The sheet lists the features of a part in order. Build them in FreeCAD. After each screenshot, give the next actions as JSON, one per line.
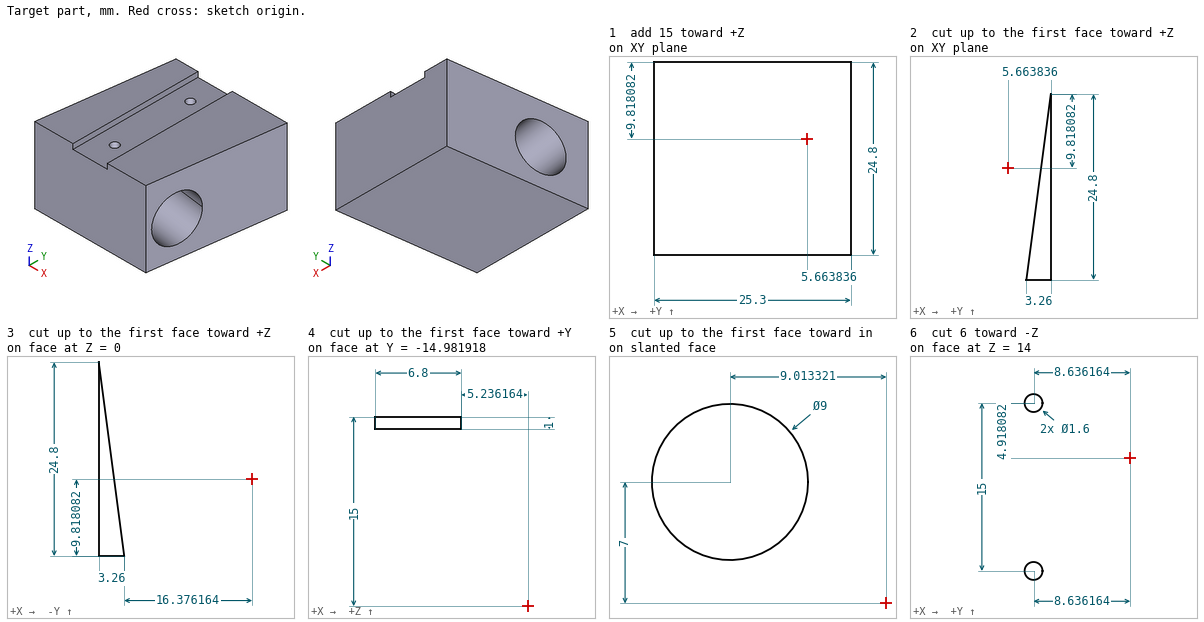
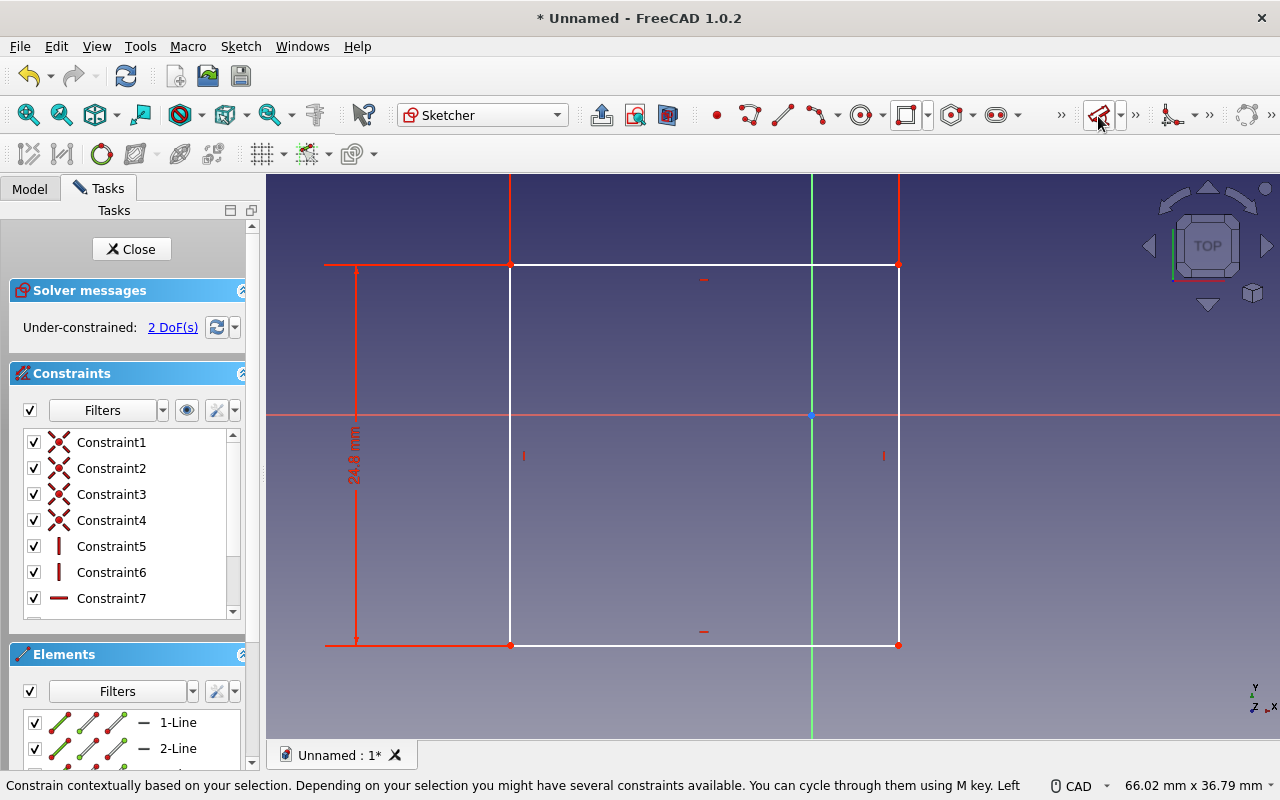
{"action": "left_click", "coordinate": [510, 265]}
{"action": "left_click", "coordinate": [476, 340]}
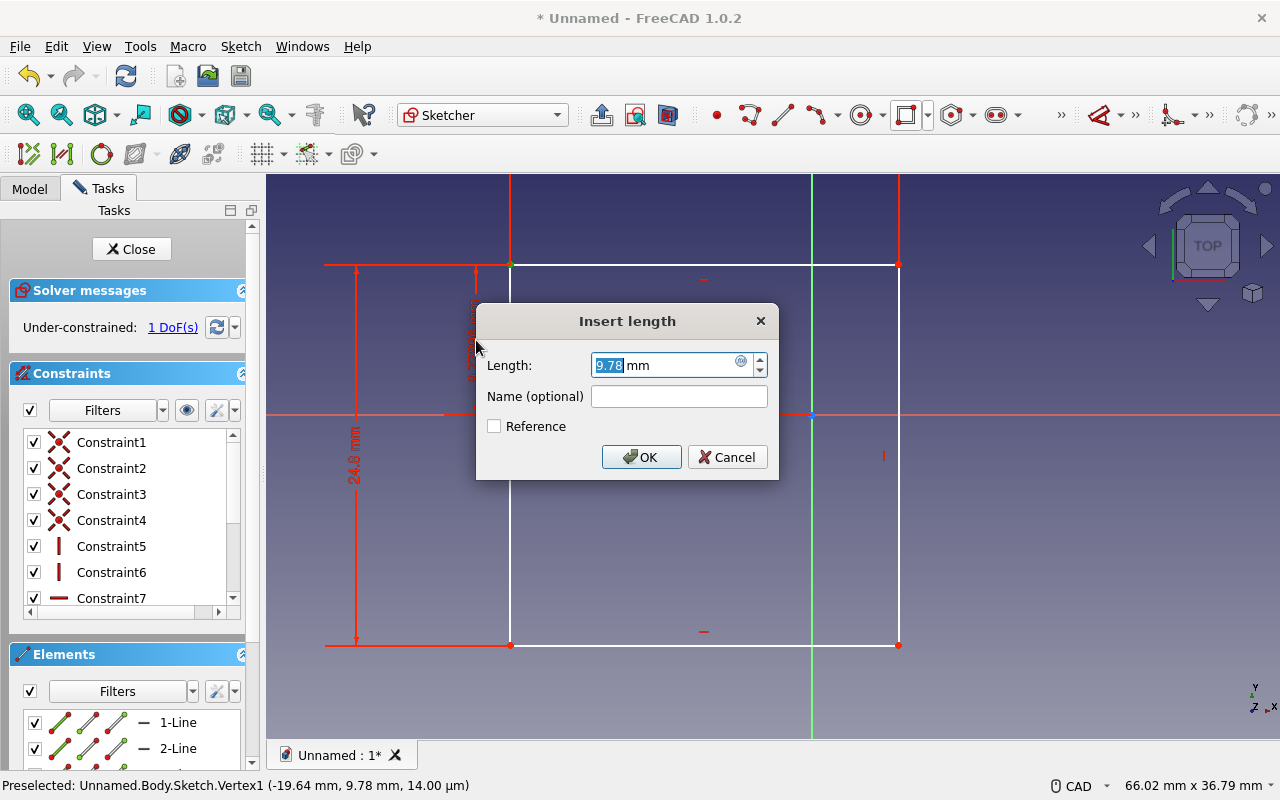
{"action": "type", "text": "9.818082"}
{"action": "key", "text": "Return"}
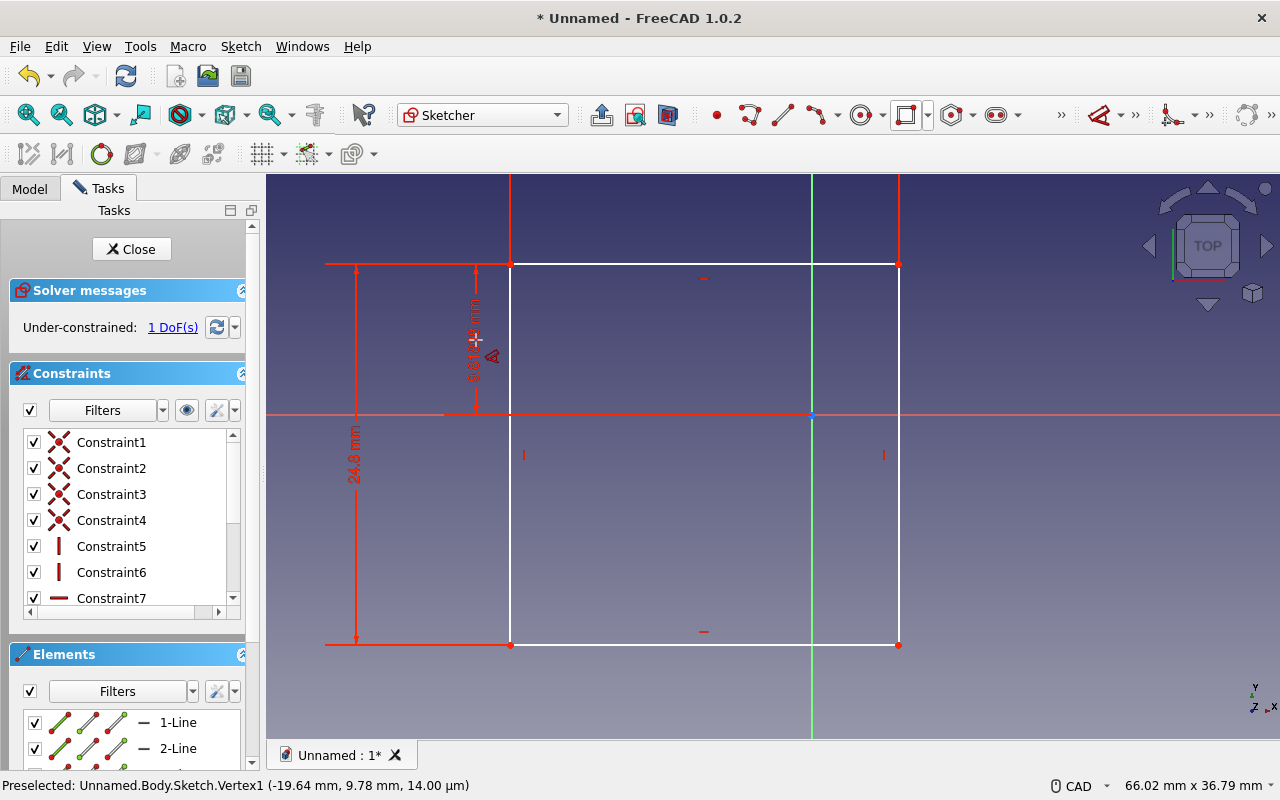
{"action": "left_click", "coordinate": [899, 645]}
{"action": "left_click", "coordinate": [855, 679]}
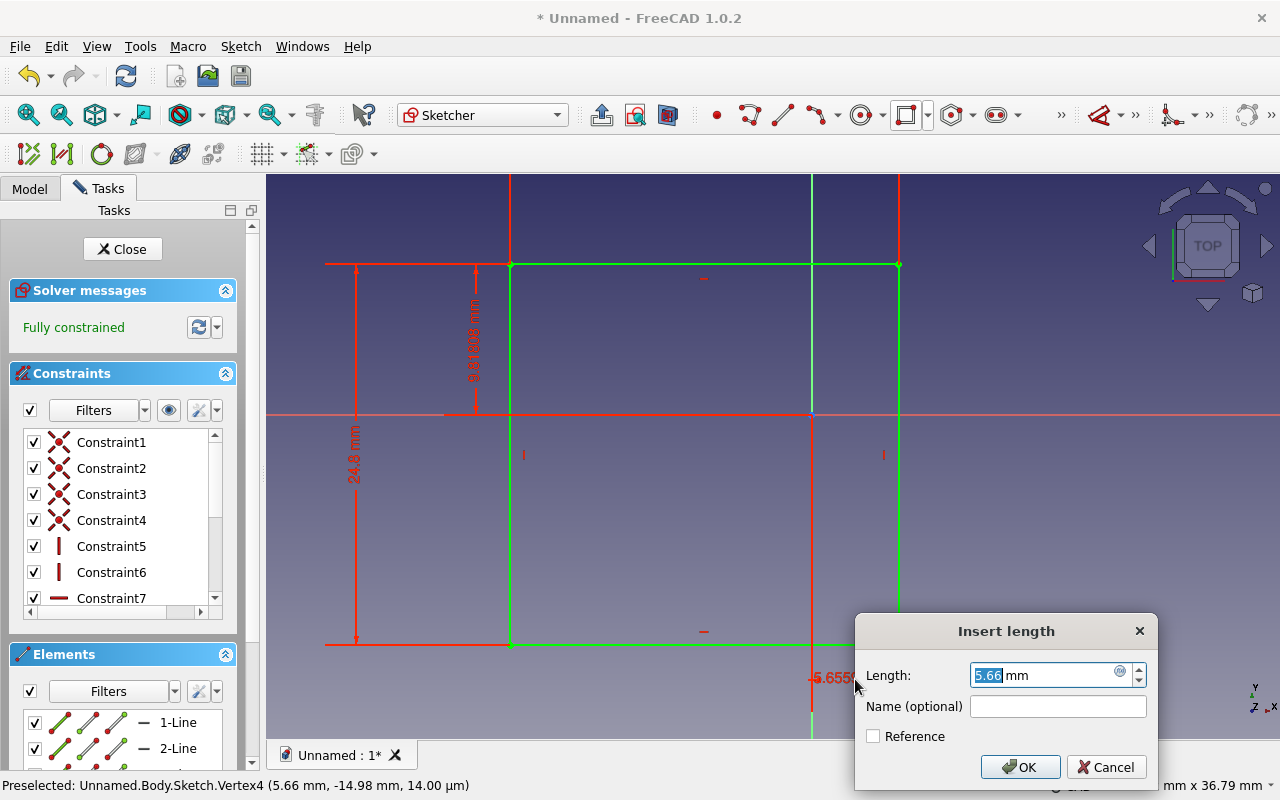
{"action": "type", "text": "5.663836"}
{"action": "key", "text": "Return"}
{"action": "key", "text": "Escape"}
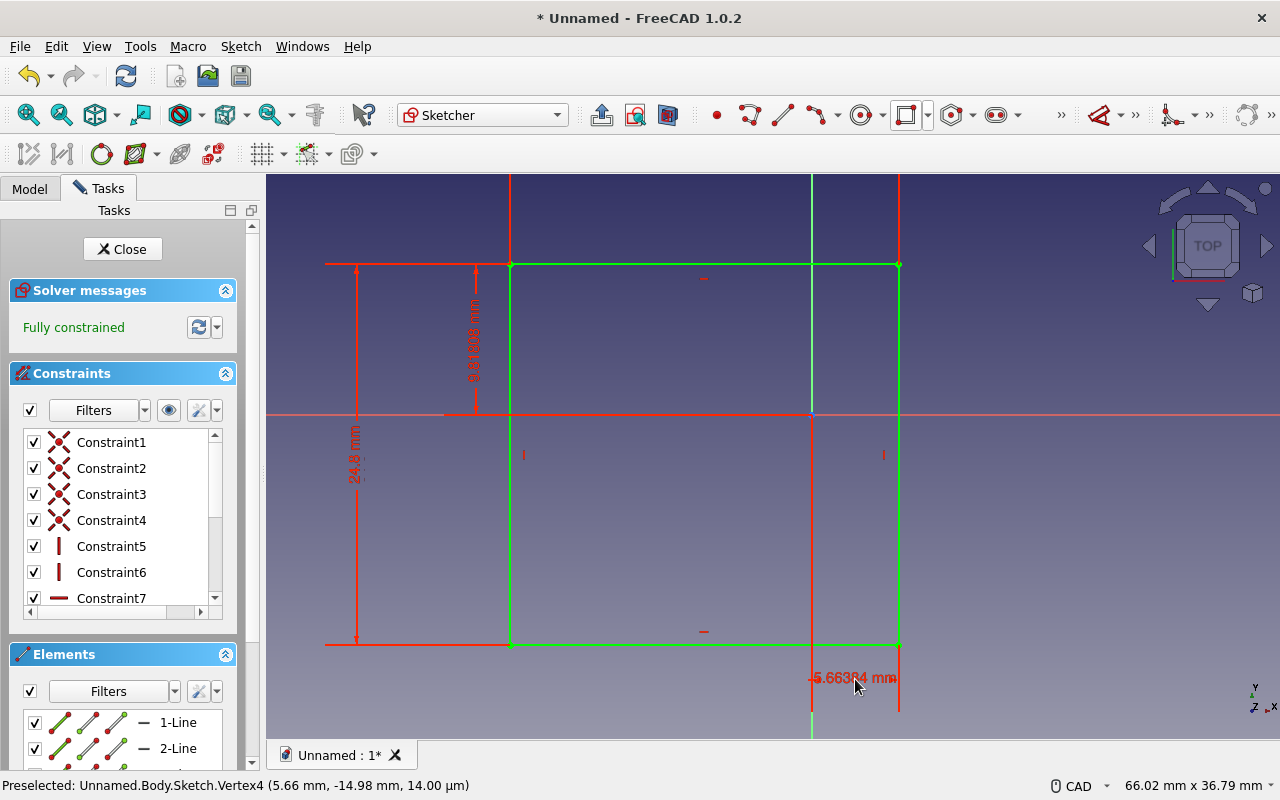
{"action": "left_click", "coordinate": [123, 249]}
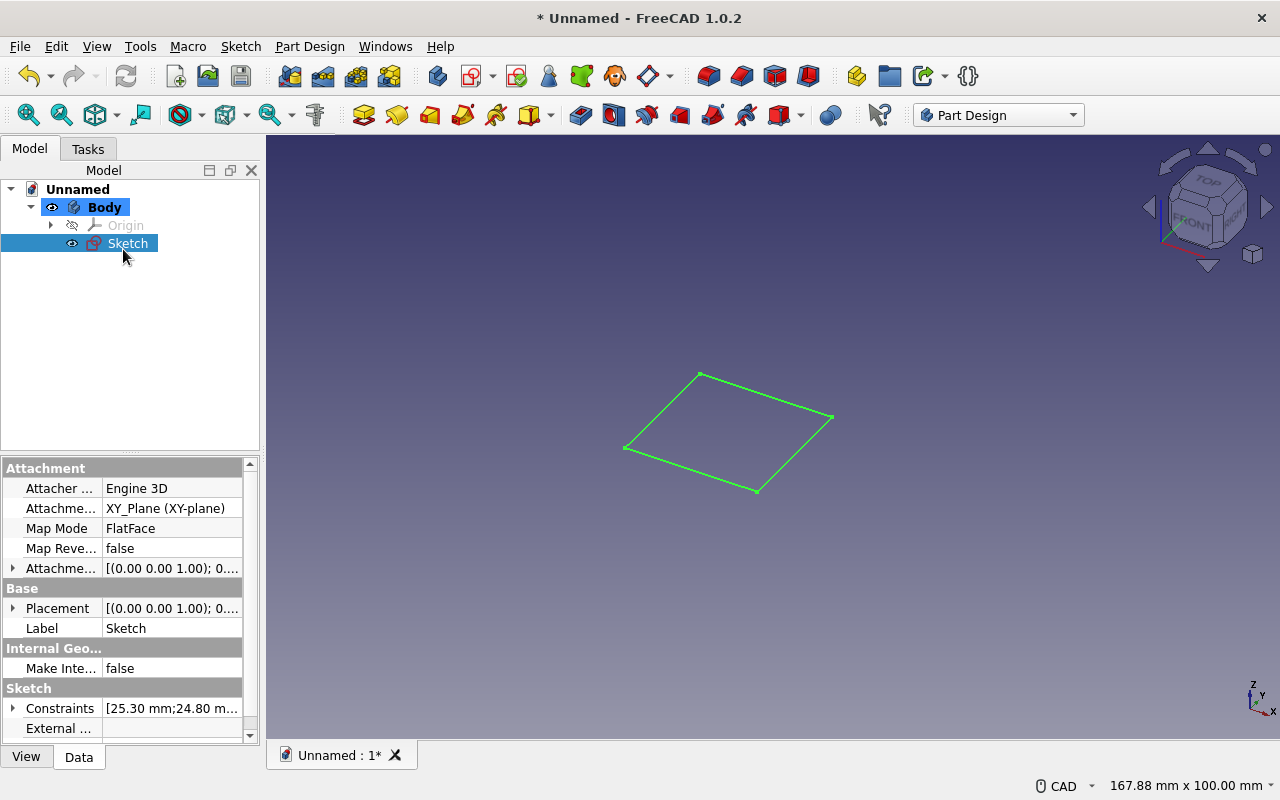
{"action": "left_click", "coordinate": [364, 116]}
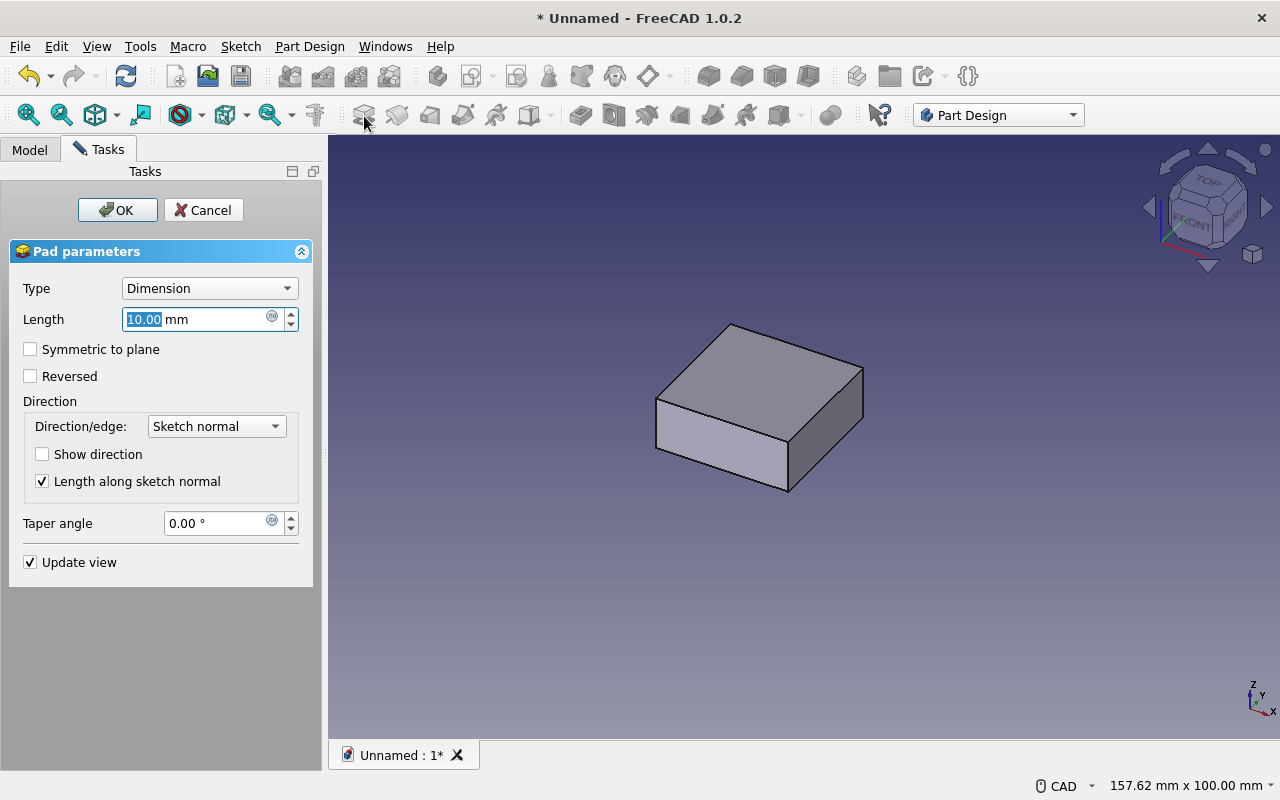
{"action": "type", "text": "15"}
{"action": "key", "text": "Tab"}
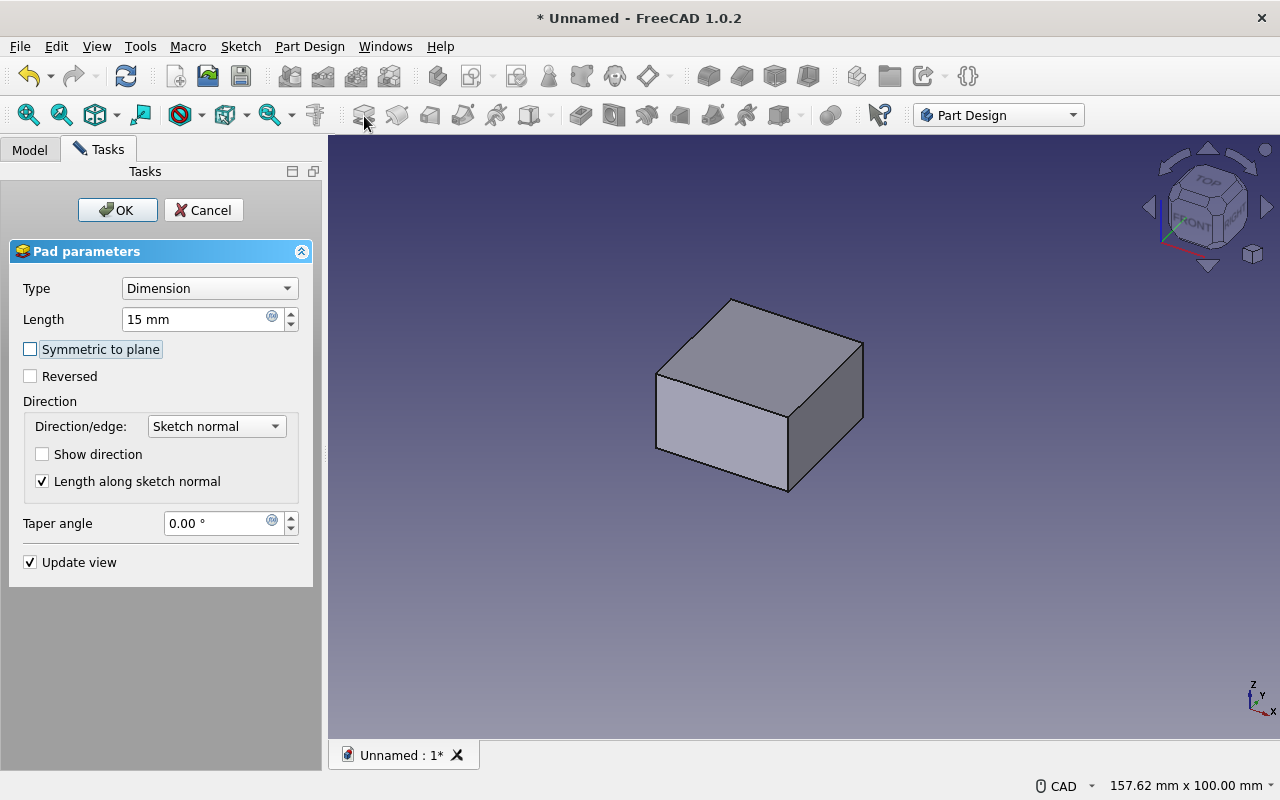
{"action": "left_click", "coordinate": [118, 210]}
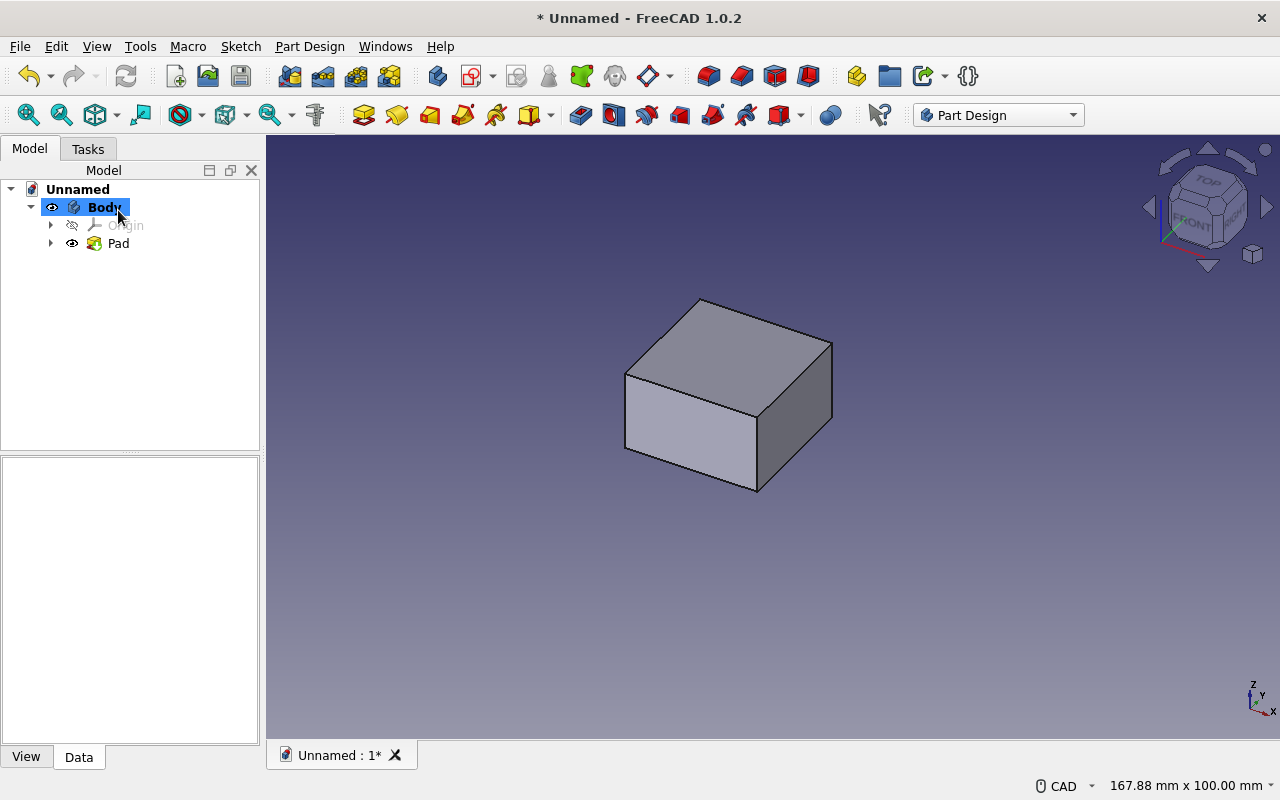
{"action": "key", "text": "v f"}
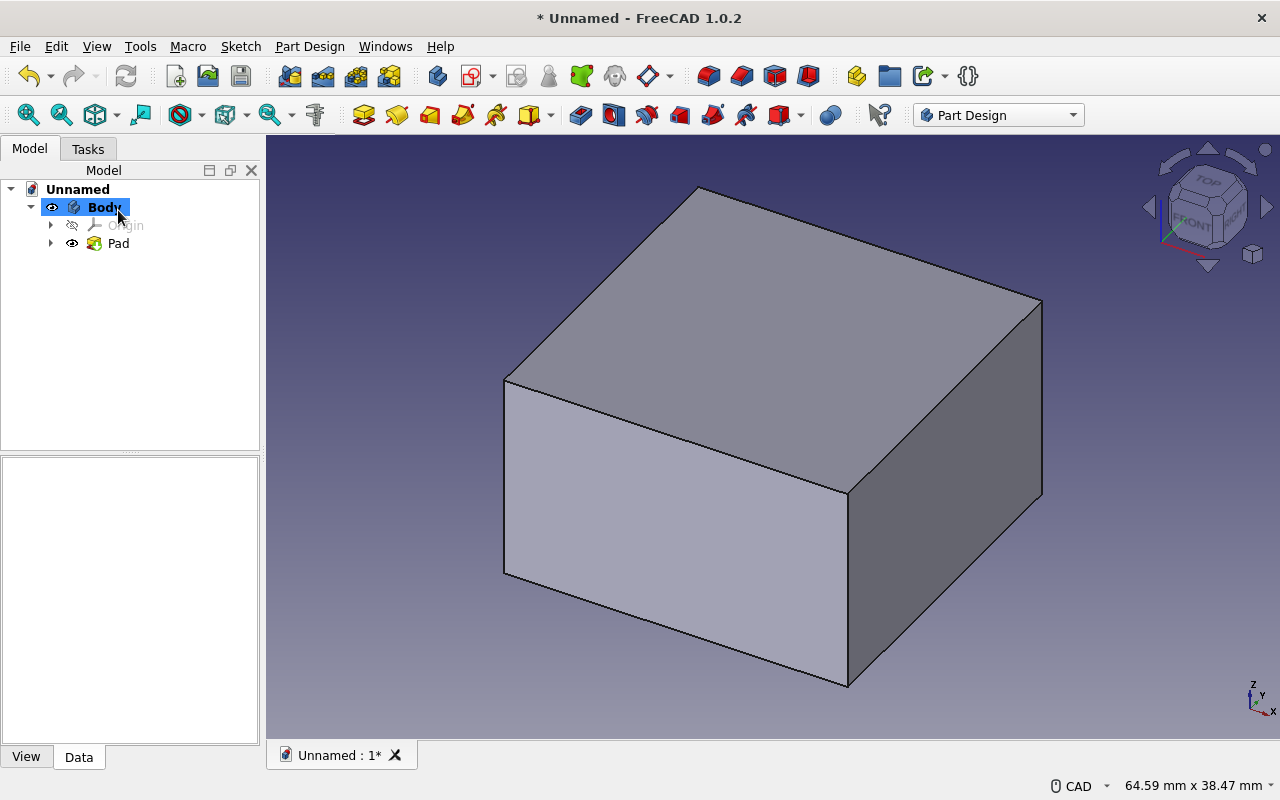
{"action": "left_click", "coordinate": [470, 76]}